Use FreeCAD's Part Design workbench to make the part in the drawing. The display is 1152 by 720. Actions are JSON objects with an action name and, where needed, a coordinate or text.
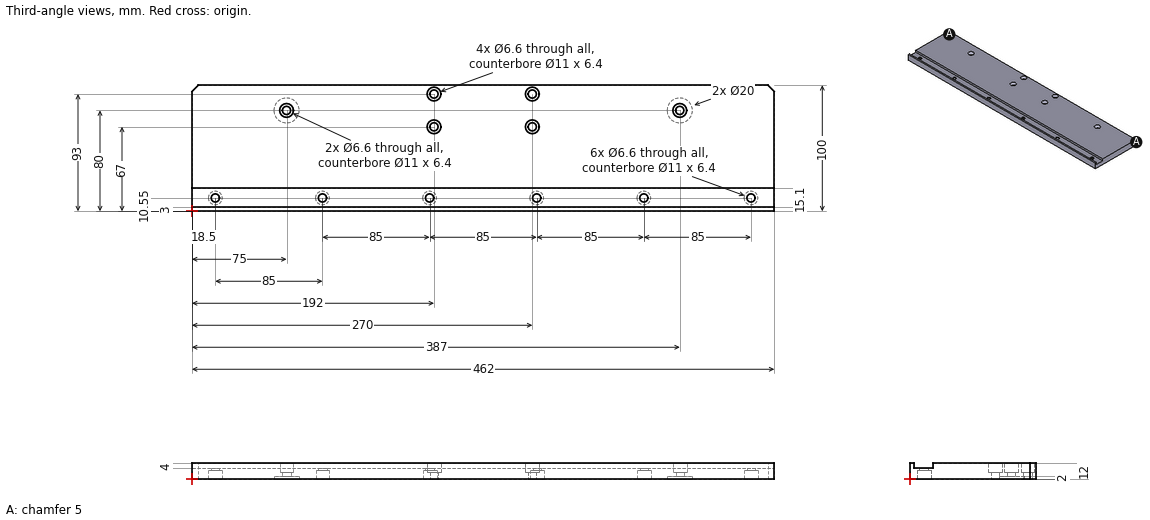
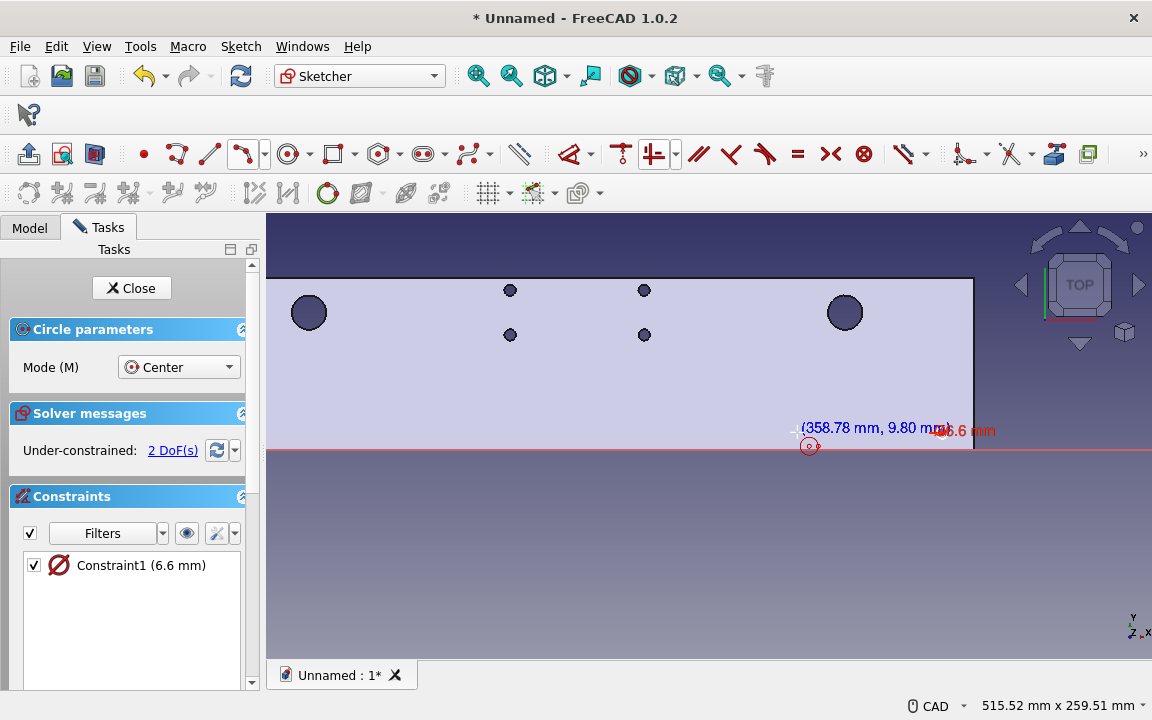
{"action": "left_click", "coordinate": [796, 432]}
{"action": "mouse_move", "coordinate": [800, 428]}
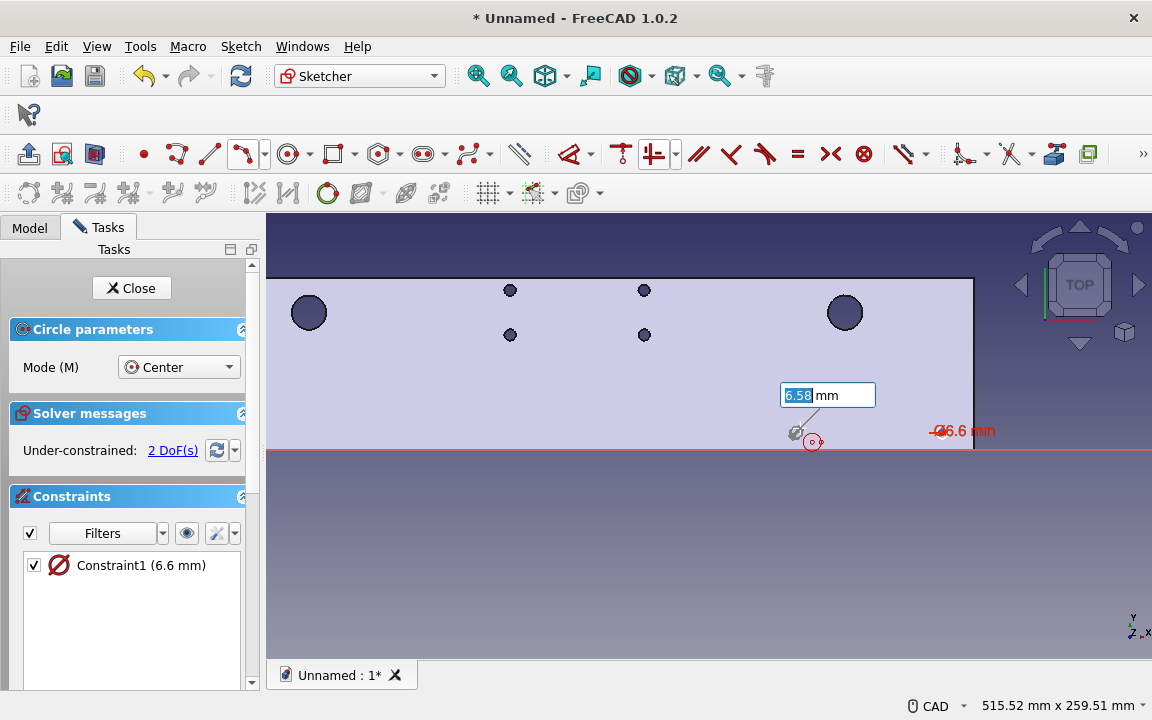
{"action": "type", "text": "6.6"}
{"action": "key", "text": "Return"}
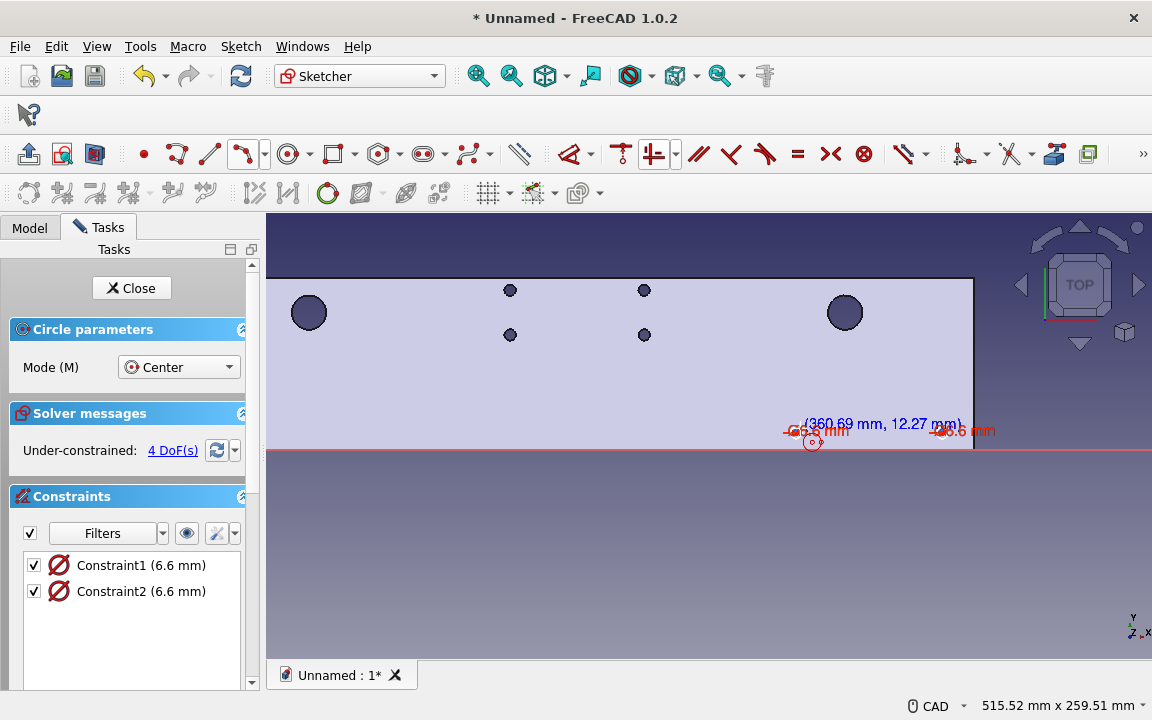
{"action": "scroll", "coordinate": [650, 432], "scroll_direction": "up", "scroll_amount": 7}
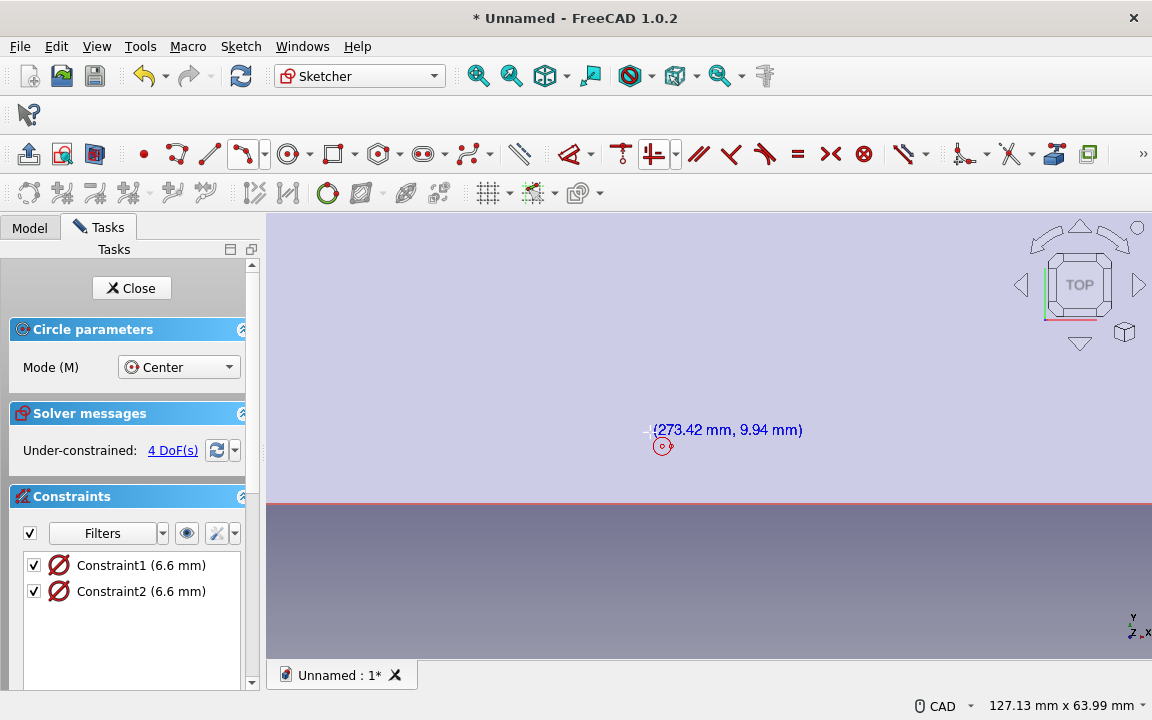
{"action": "scroll", "coordinate": [708, 432], "scroll_direction": "down", "scroll_amount": 9}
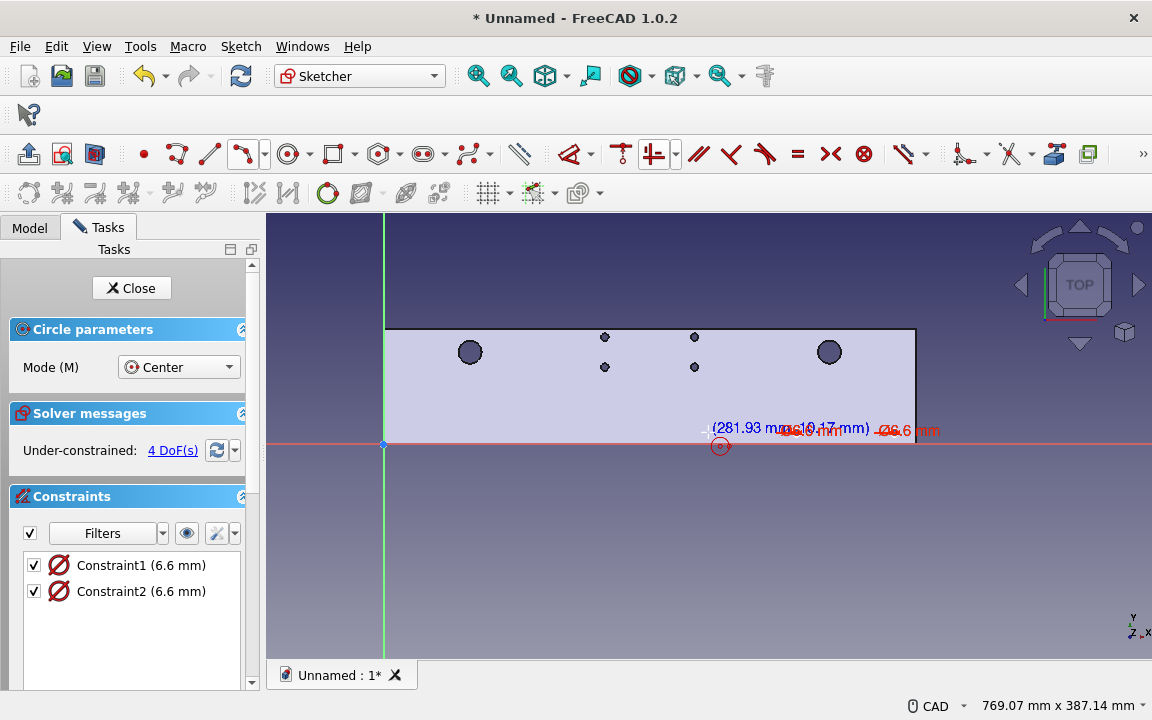
{"action": "scroll", "coordinate": [699, 432], "scroll_direction": "up", "scroll_amount": 2}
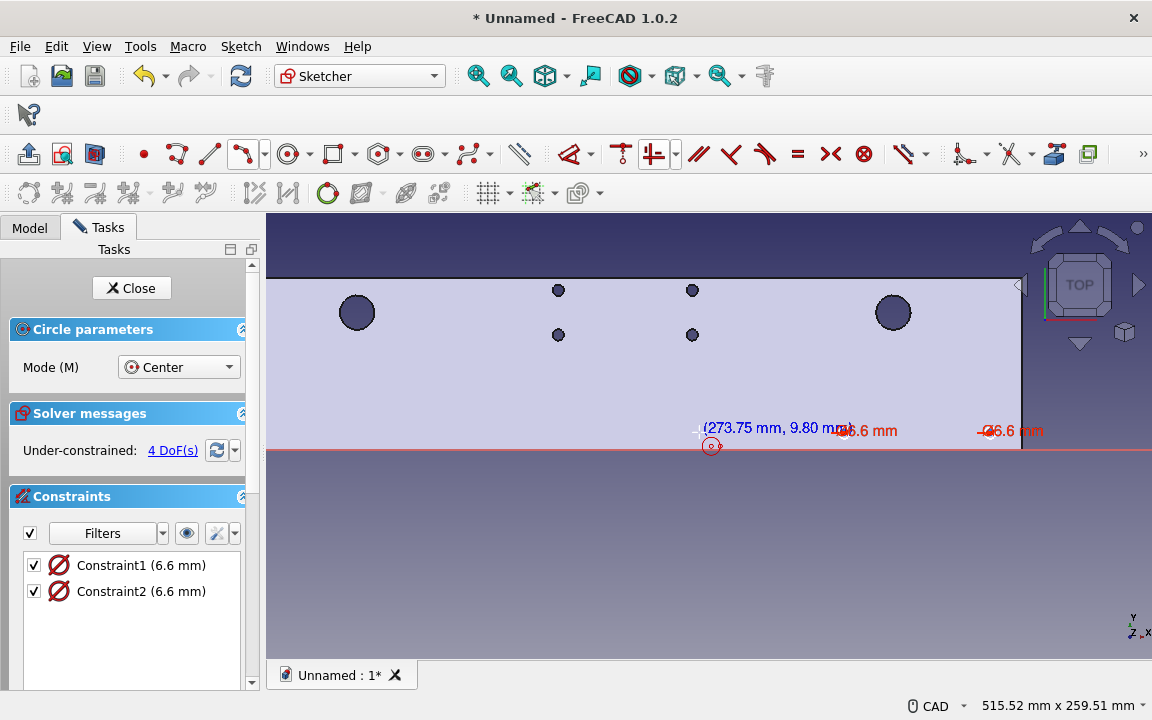
{"action": "left_click", "coordinate": [698, 432]}
{"action": "mouse_move", "coordinate": [702, 428]}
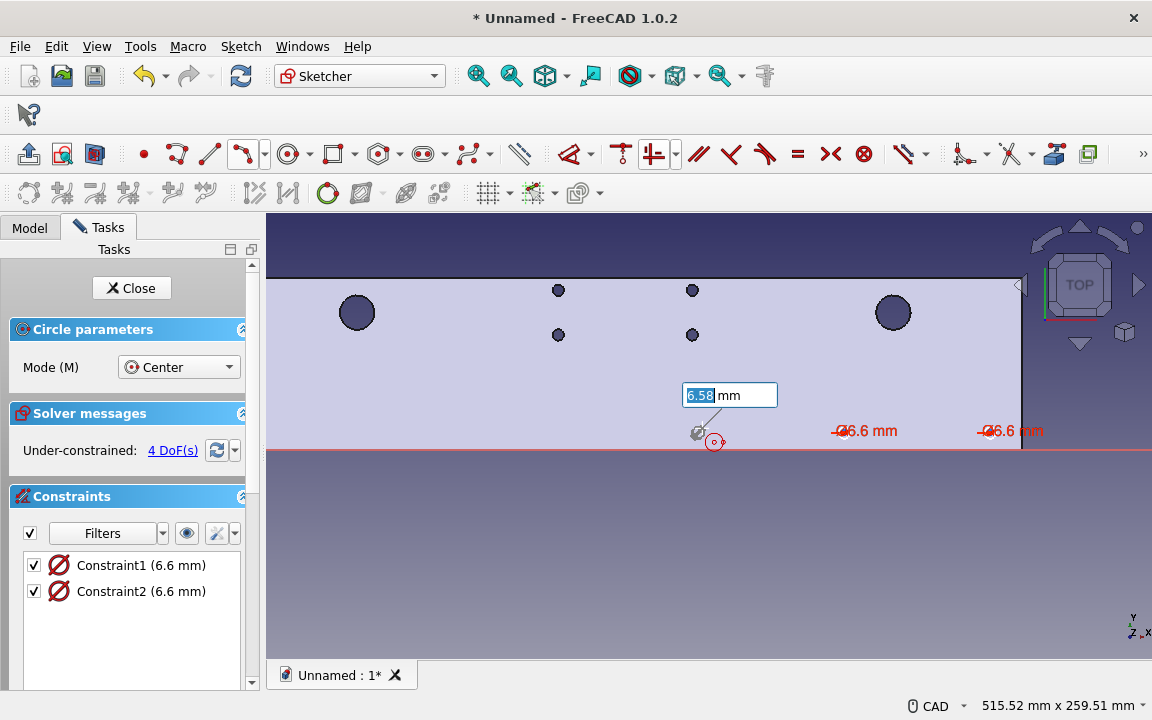
{"action": "type", "text": "6.6"}
{"action": "key", "text": "Return"}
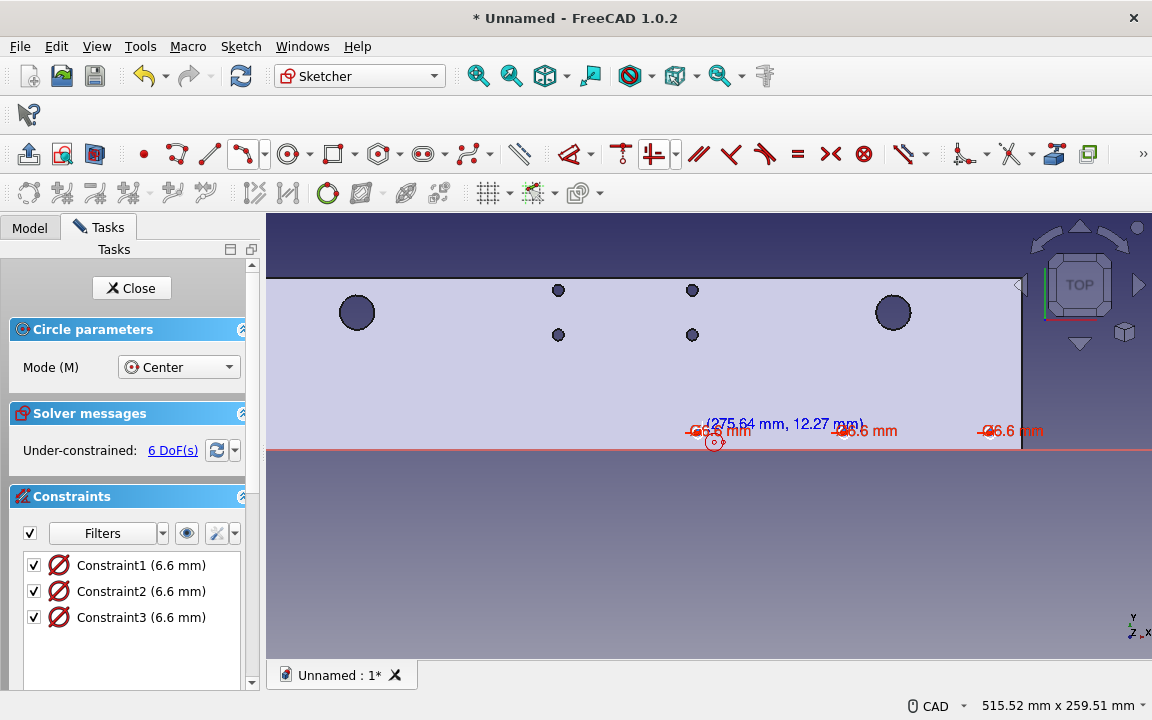
{"action": "scroll", "coordinate": [552, 432], "scroll_direction": "up", "scroll_amount": 7}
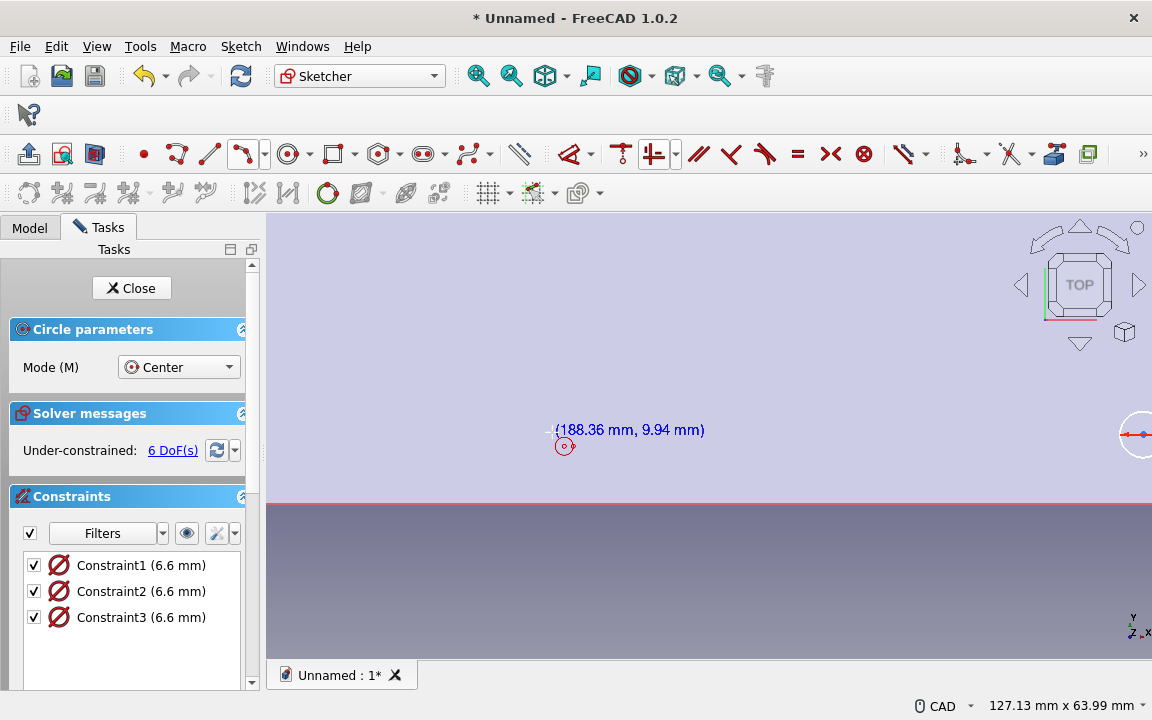
{"action": "scroll", "coordinate": [610, 432], "scroll_direction": "down", "scroll_amount": 9}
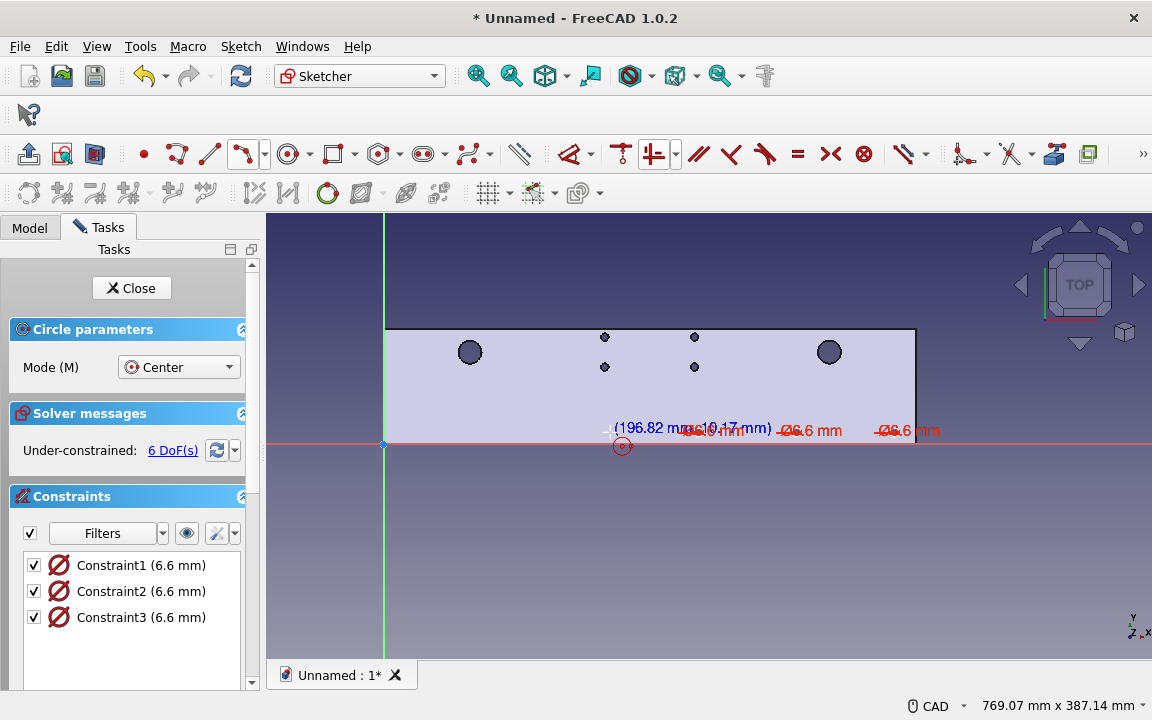
{"action": "scroll", "coordinate": [601, 432], "scroll_direction": "up", "scroll_amount": 2}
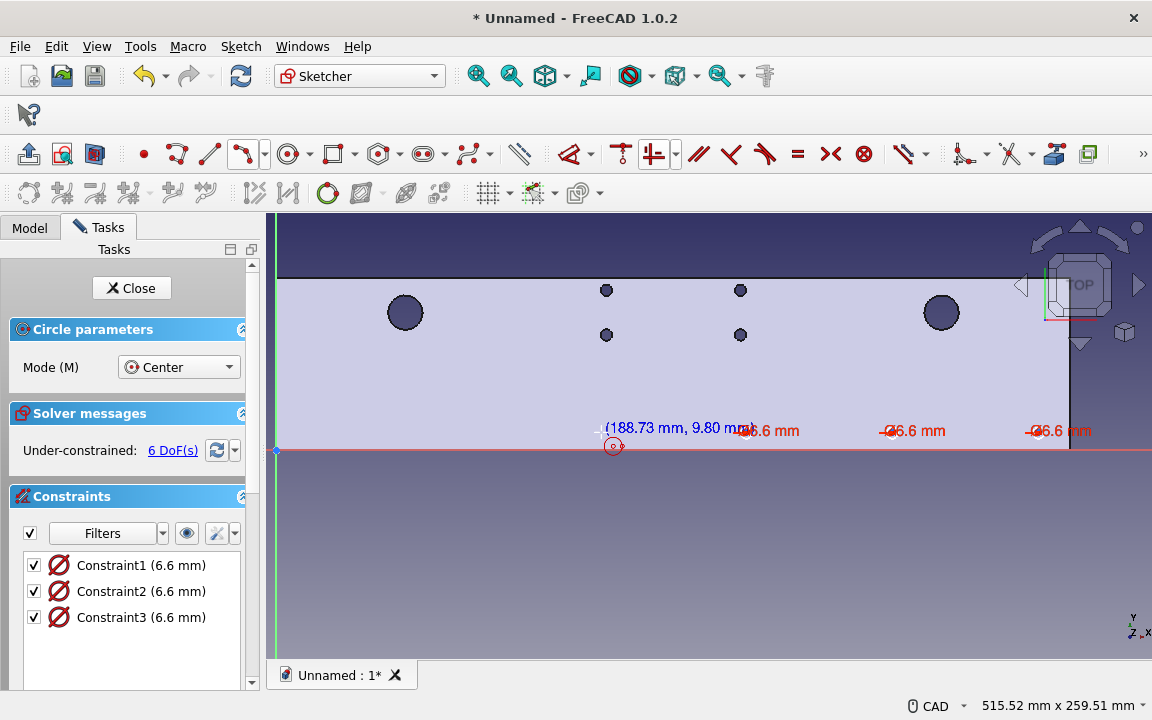
{"action": "left_click", "coordinate": [600, 432]}
{"action": "mouse_move", "coordinate": [604, 428]}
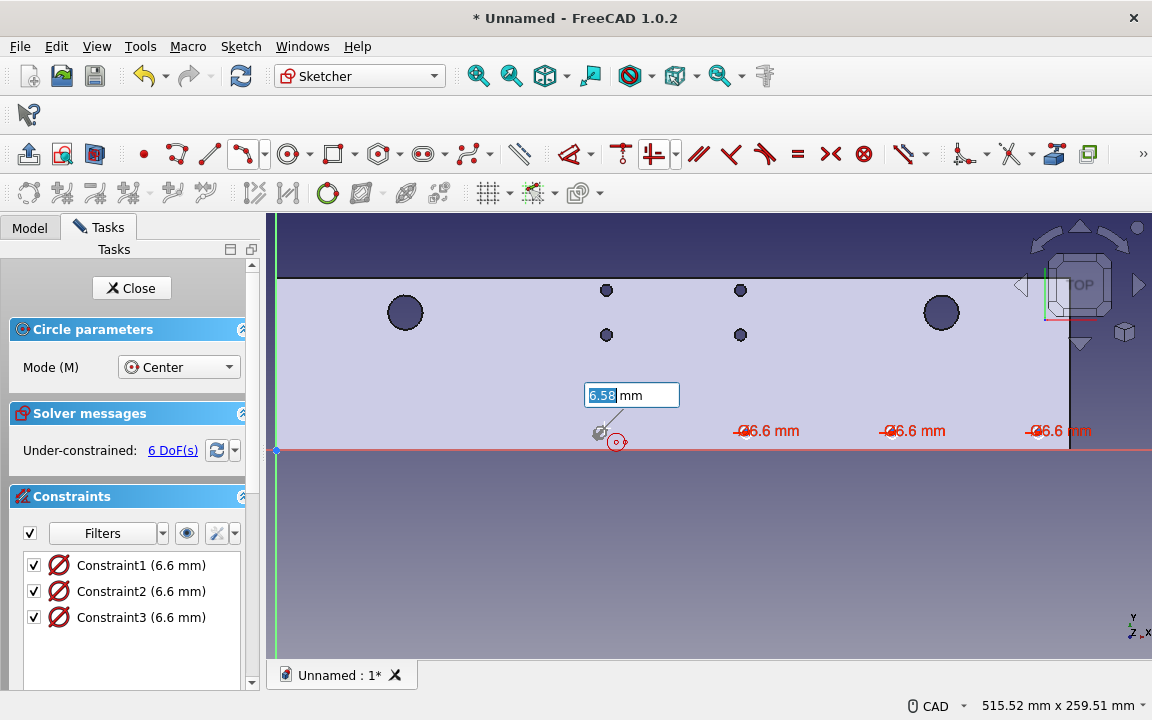
{"action": "type", "text": "6.6"}
{"action": "key", "text": "Return"}